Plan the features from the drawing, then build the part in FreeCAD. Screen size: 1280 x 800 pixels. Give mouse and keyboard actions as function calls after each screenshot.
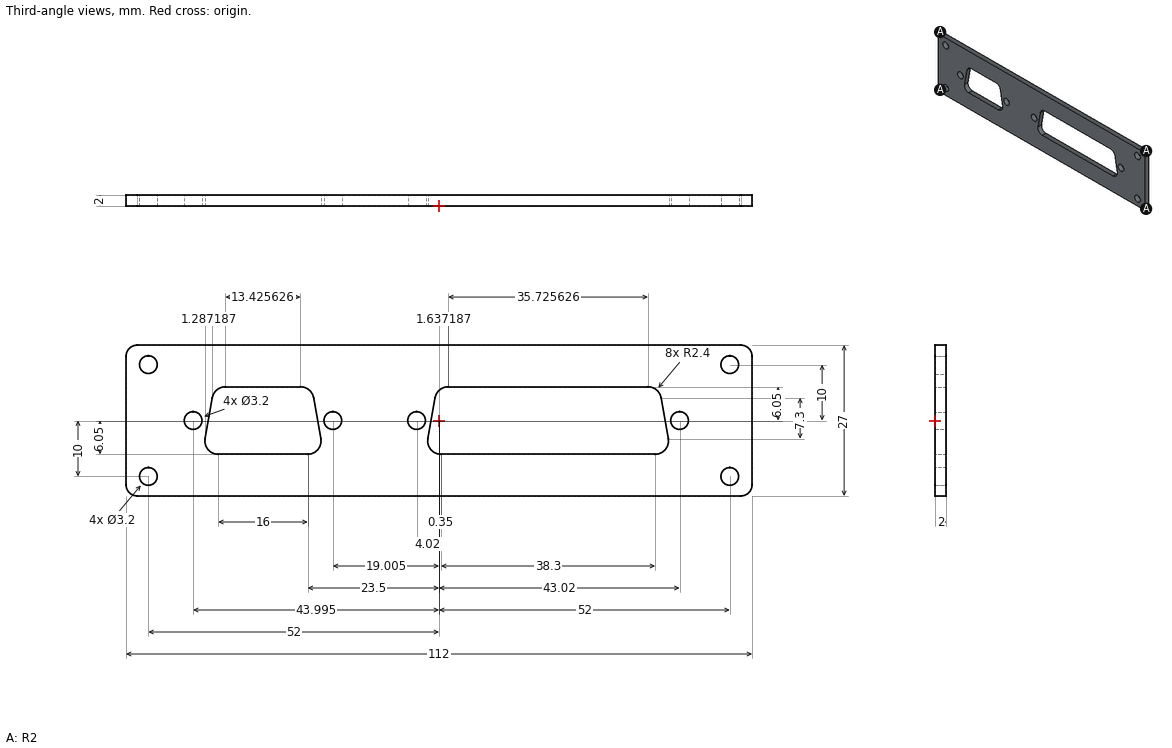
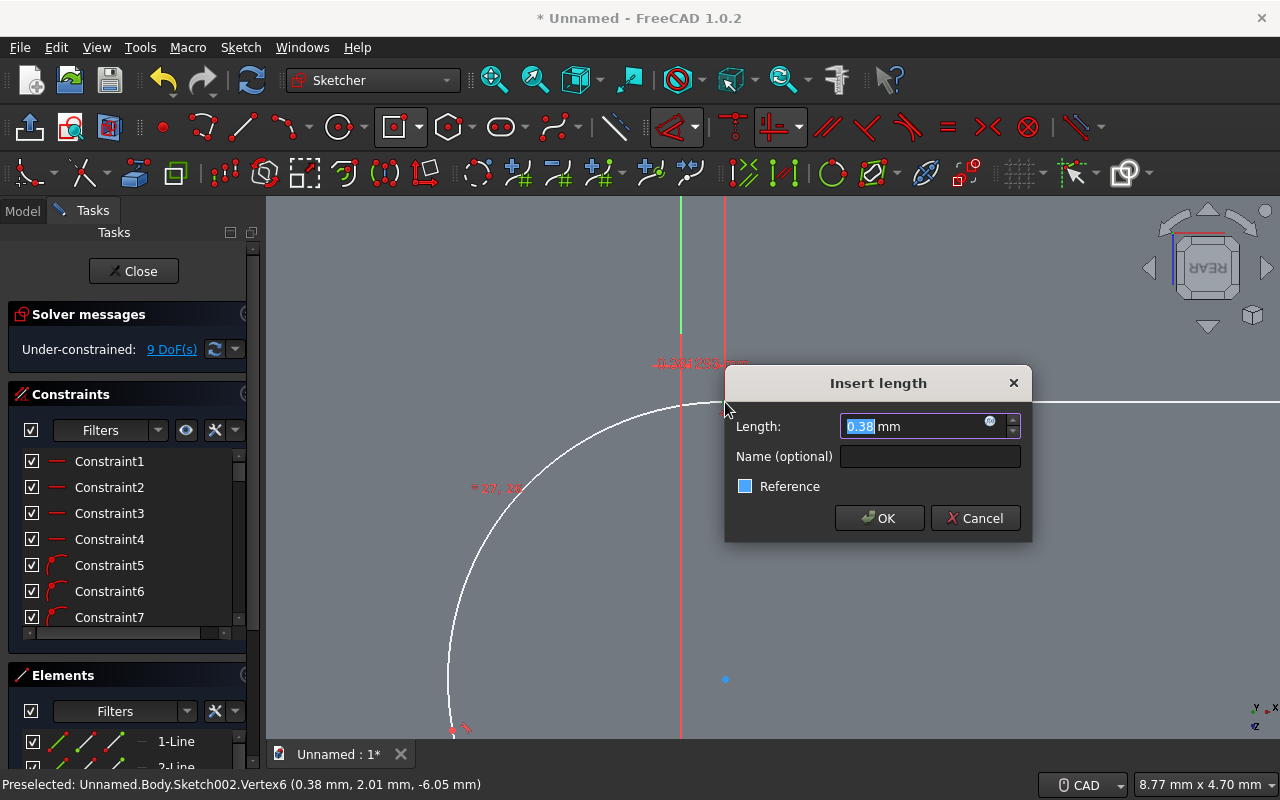
text(0.35)
key(Return)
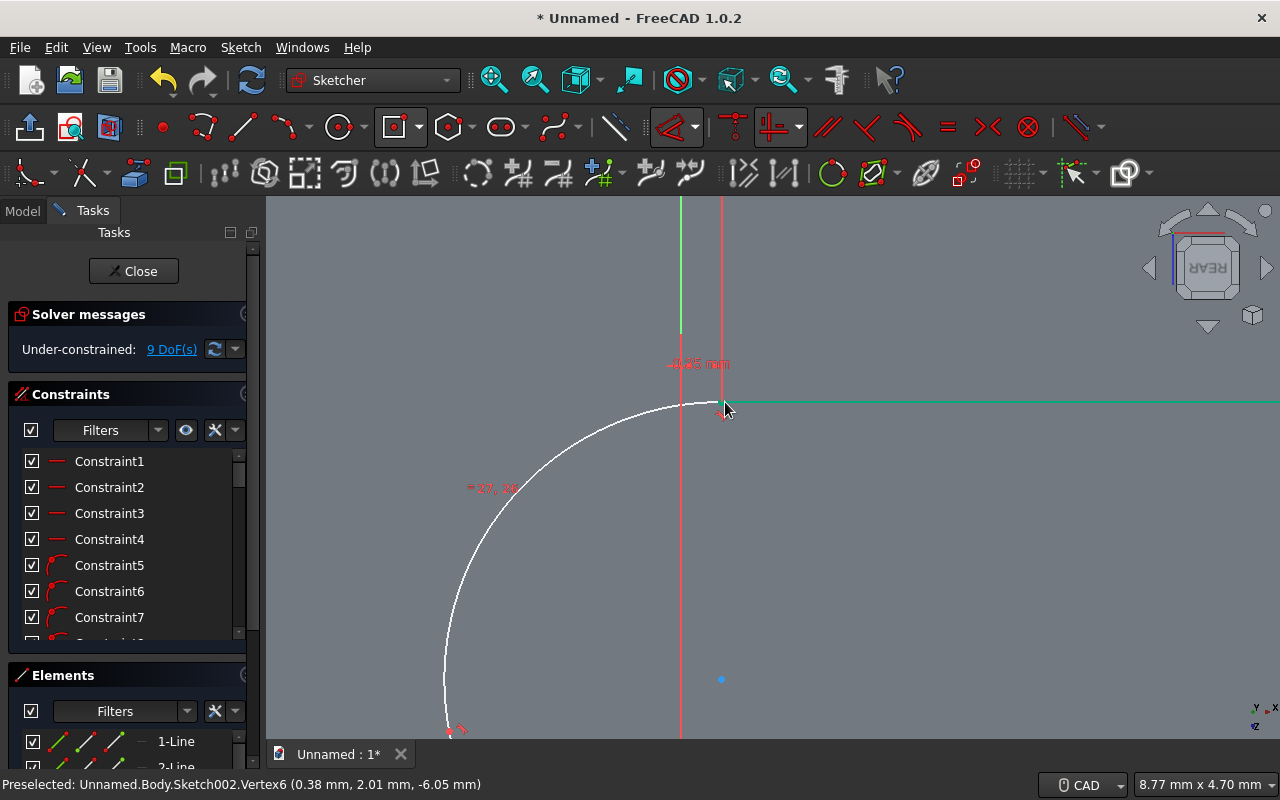
scroll(710, 426, down, 14)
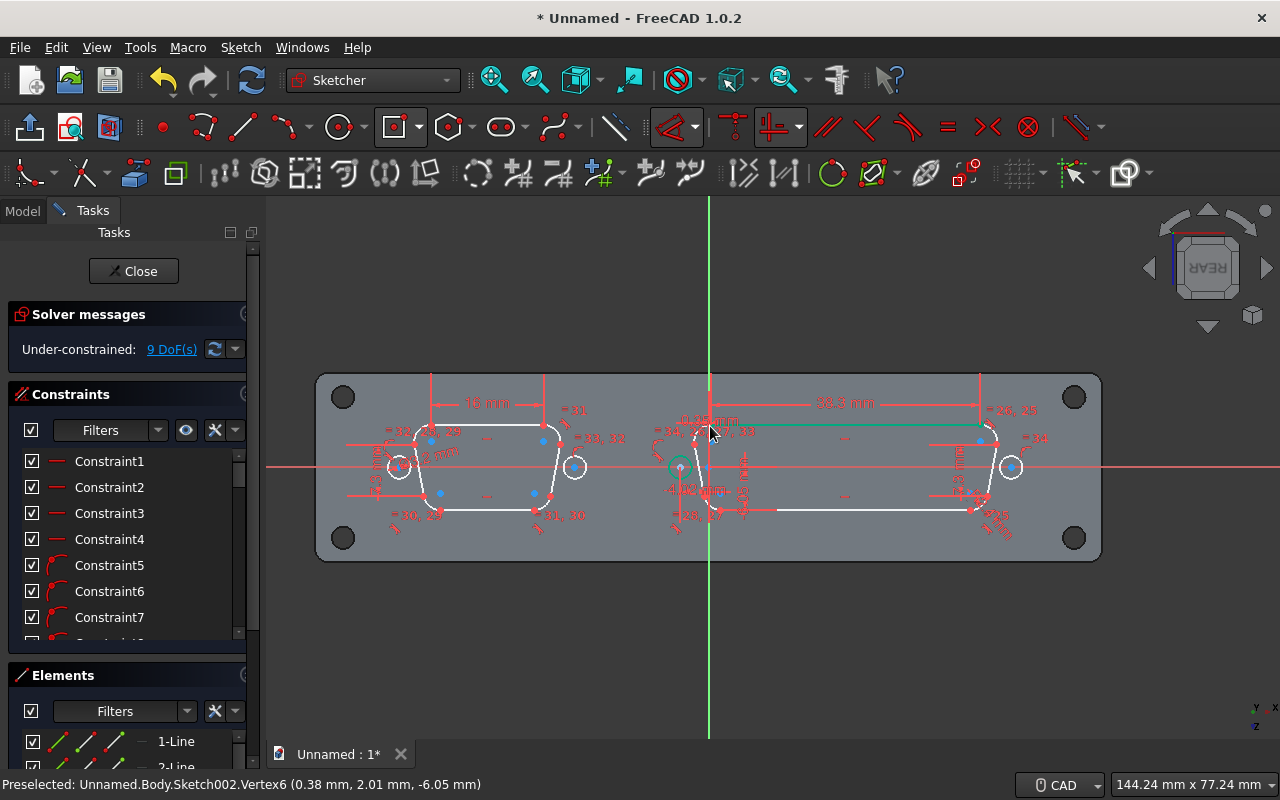
click(544, 425)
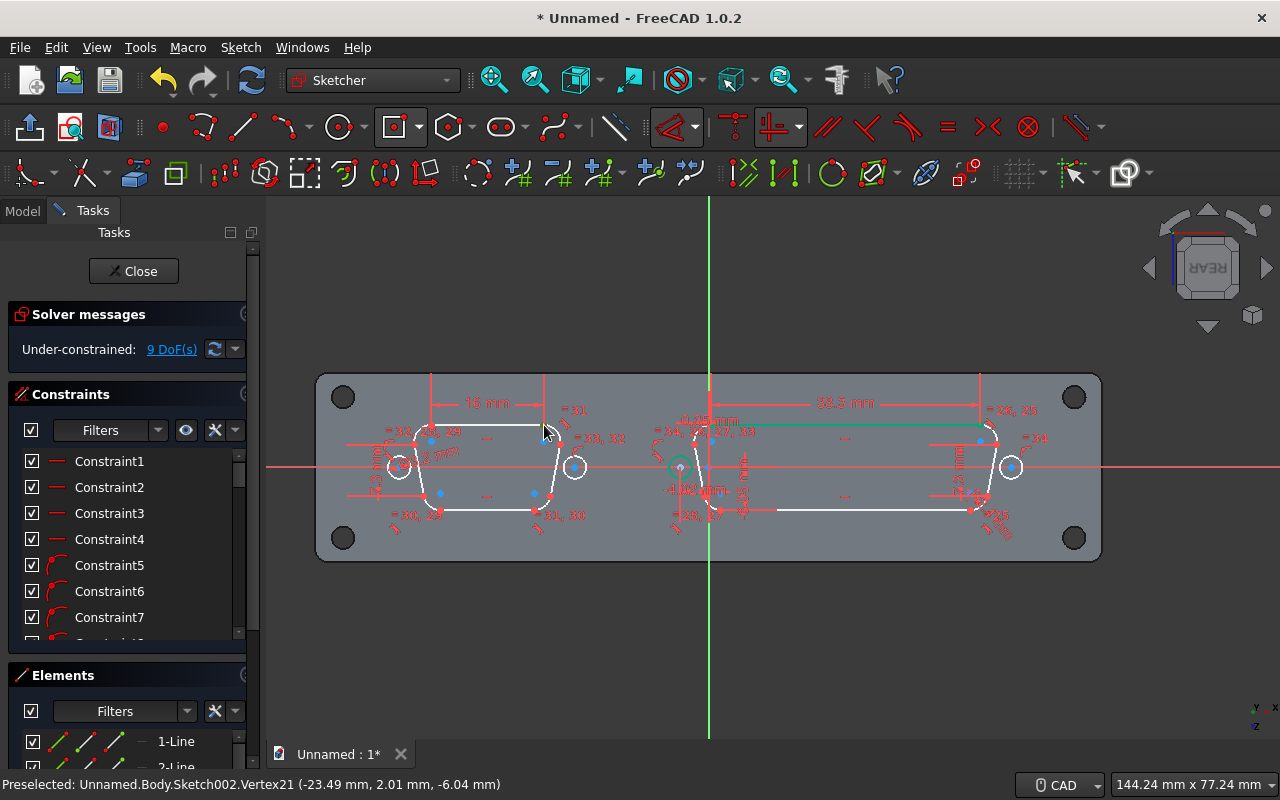
click(698, 128)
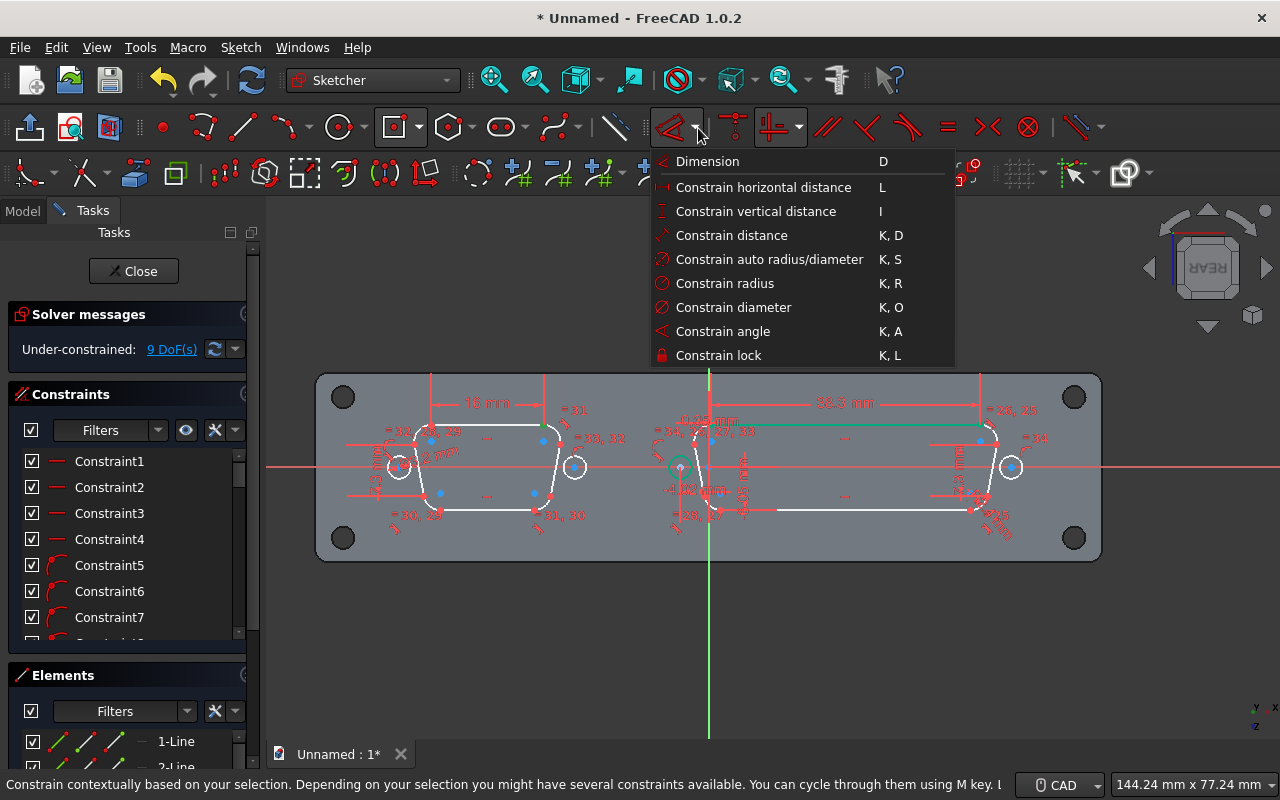
click(803, 187)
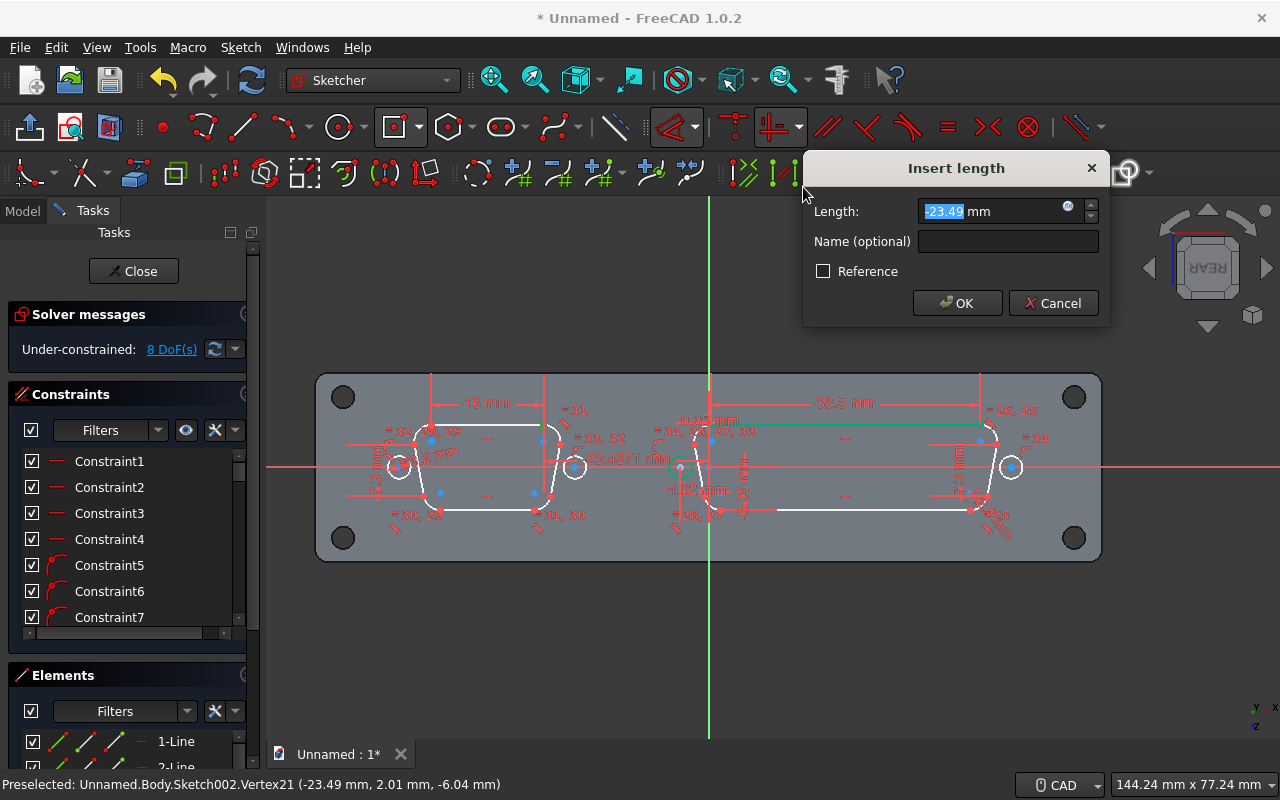
text(-23.5)
key(Return)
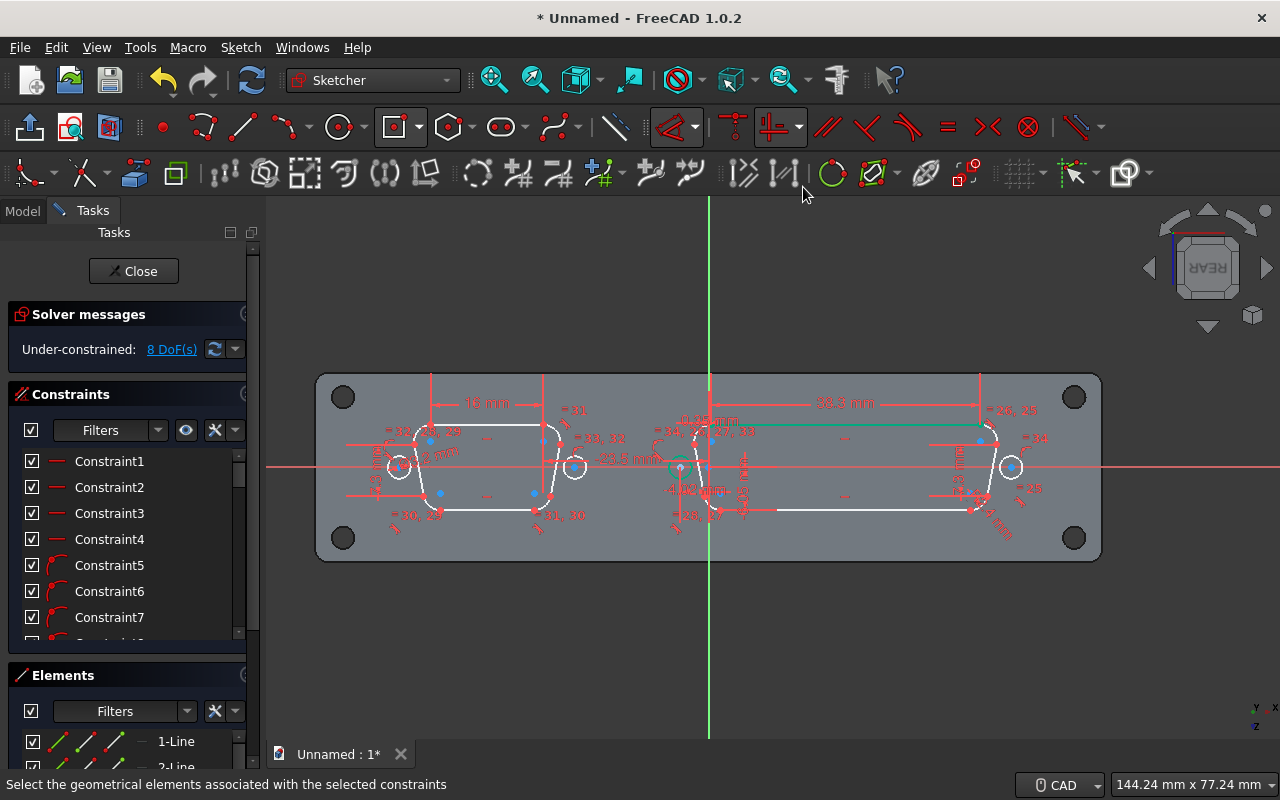
click(543, 425)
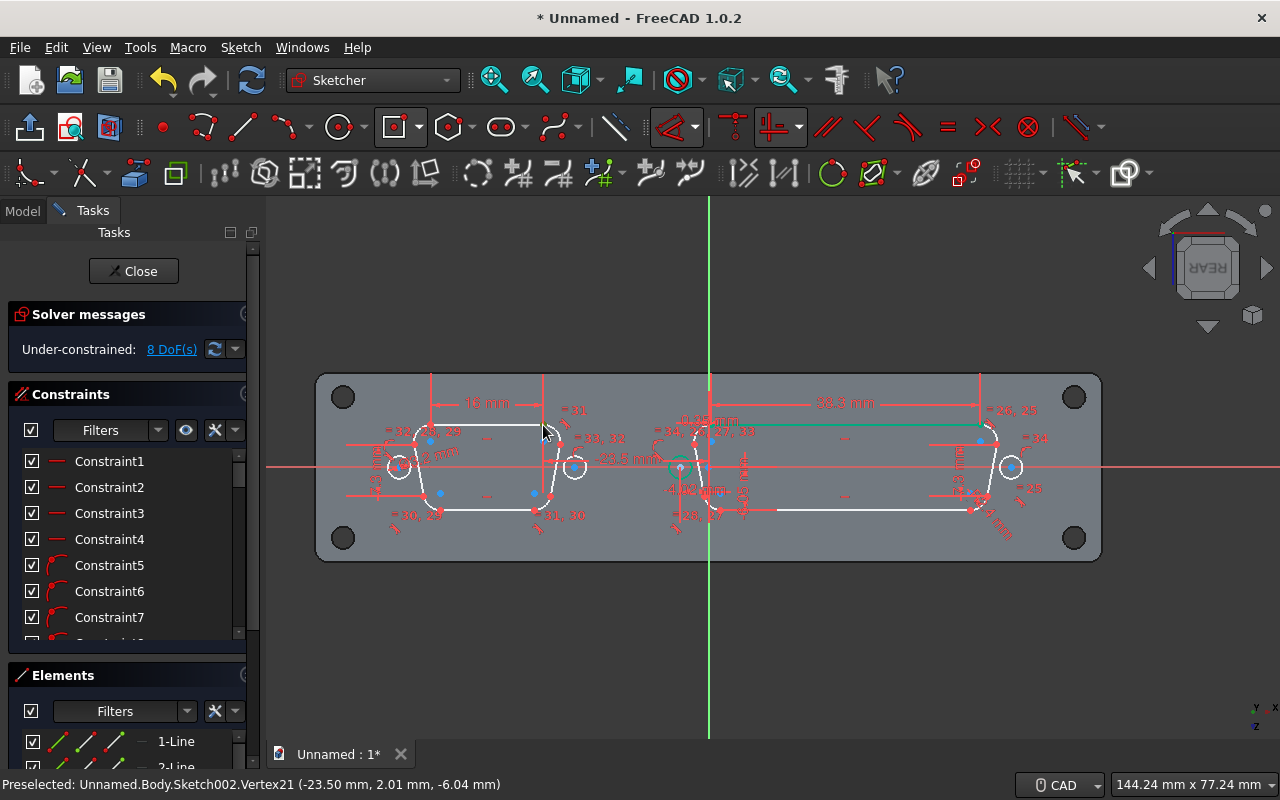
key(i)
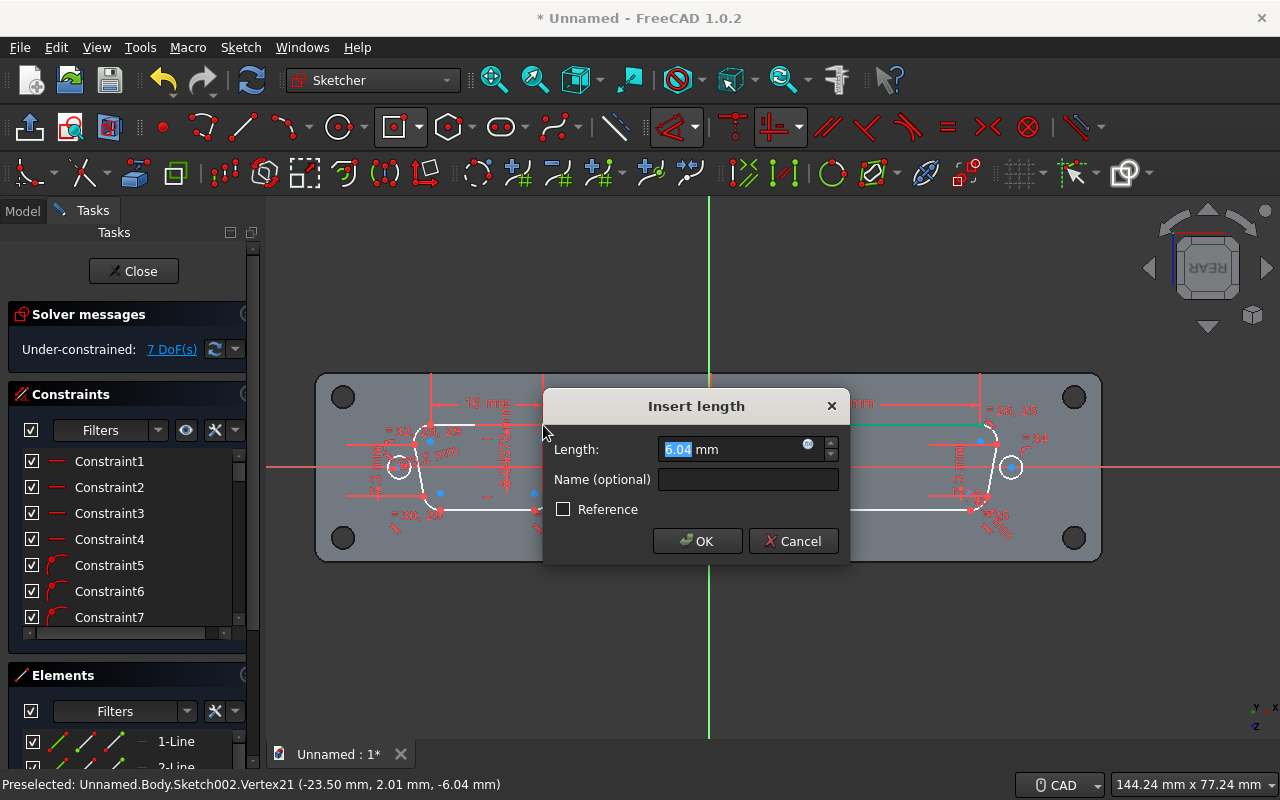
text(6.05)
key(Return)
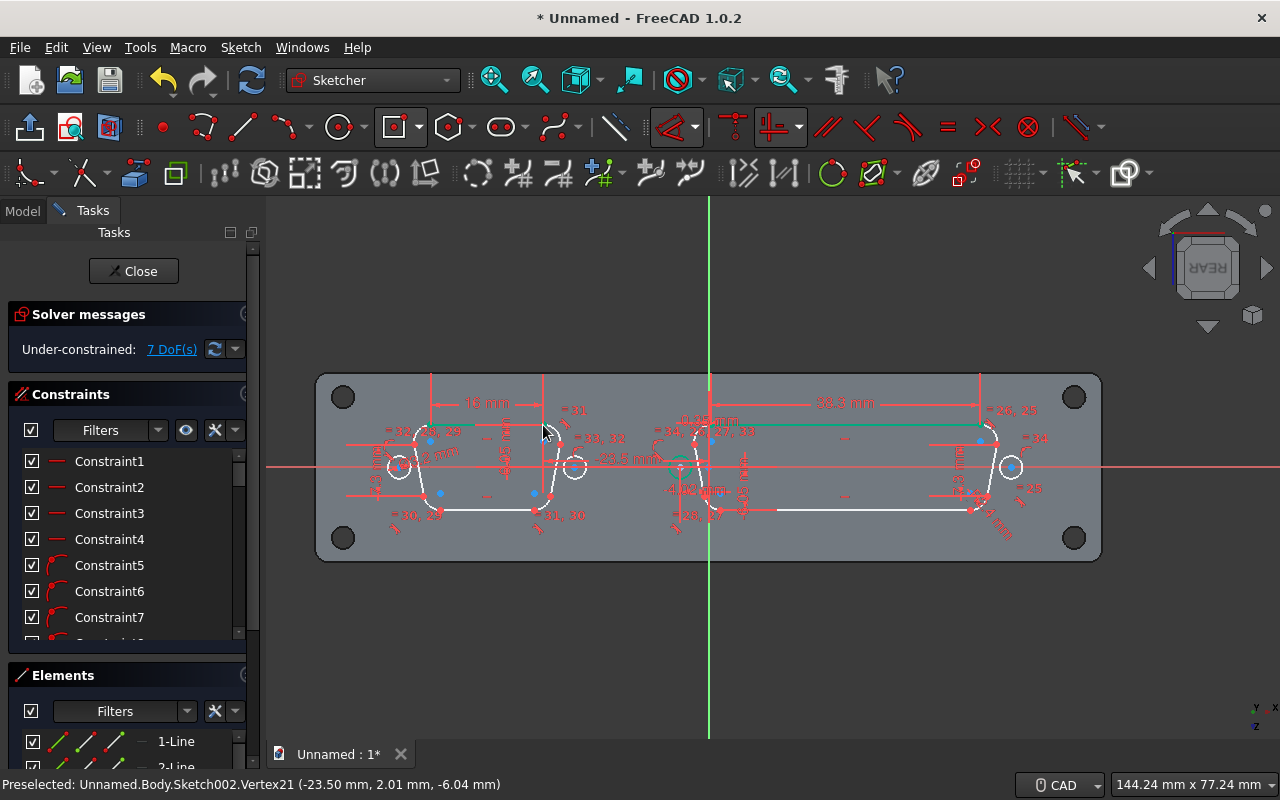
click(1011, 467)